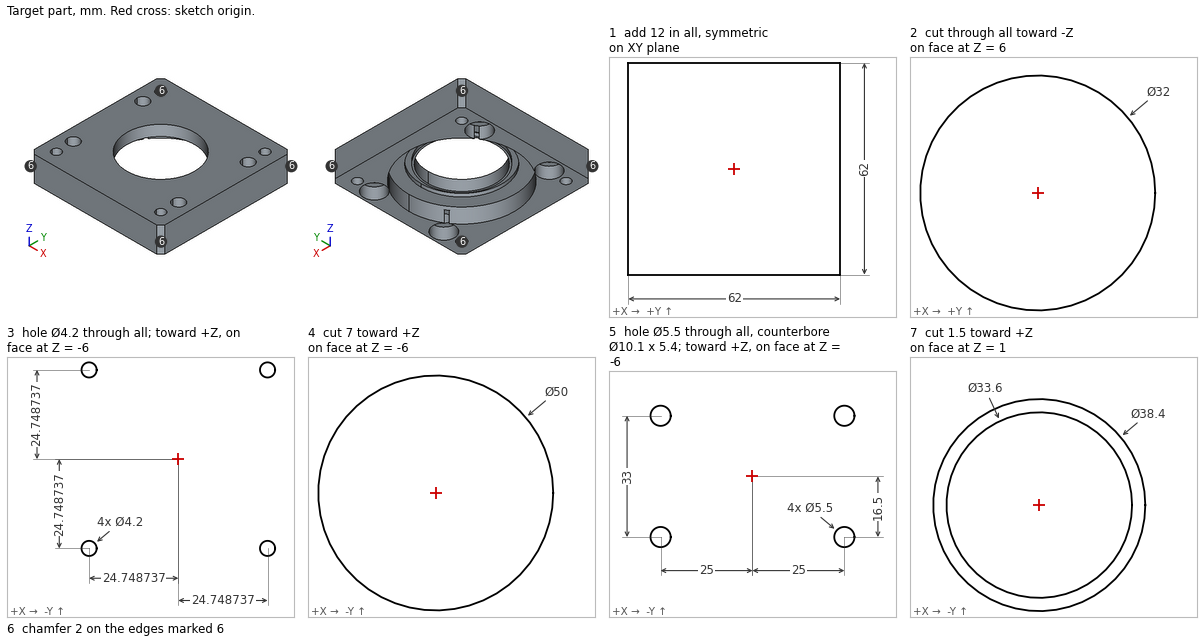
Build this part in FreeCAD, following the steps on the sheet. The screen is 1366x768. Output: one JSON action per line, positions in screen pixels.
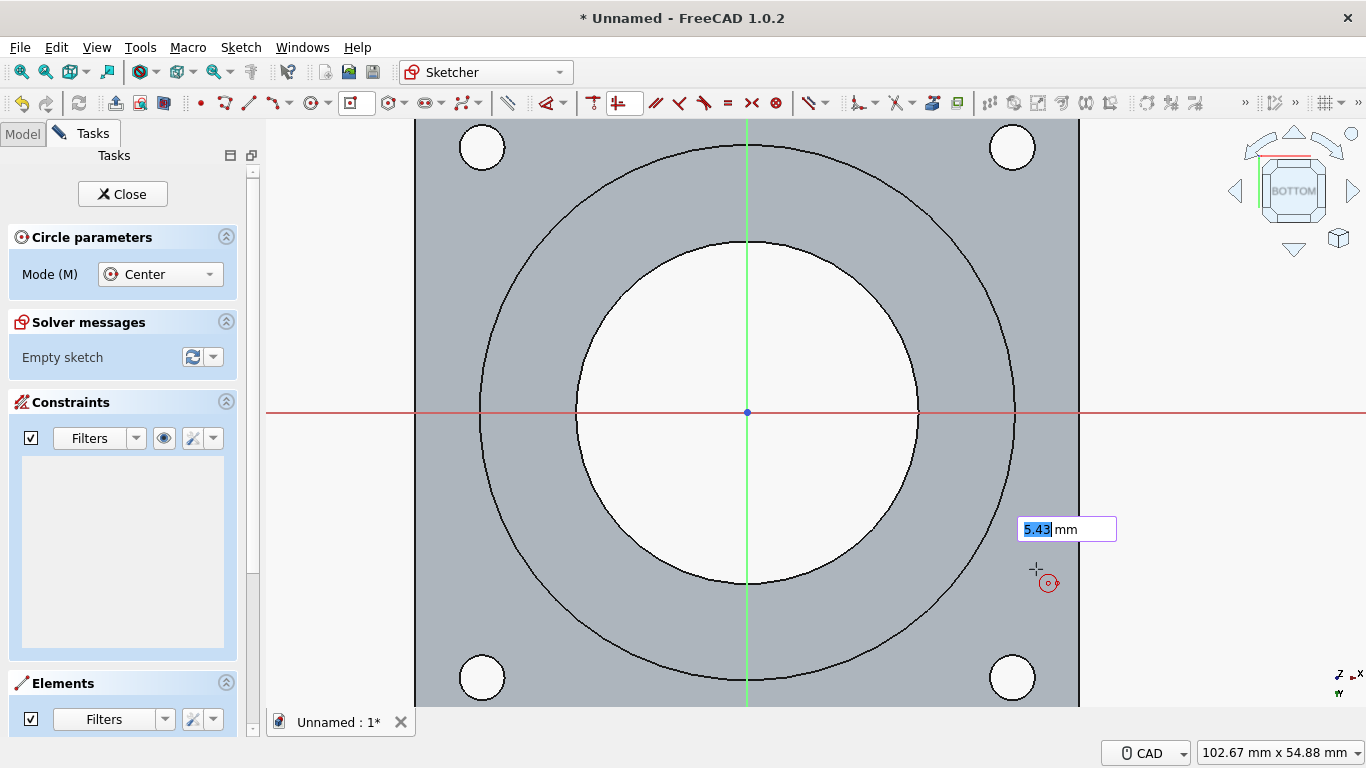
{"action": "type", "text": "5.5"}
{"action": "key", "text": "Return"}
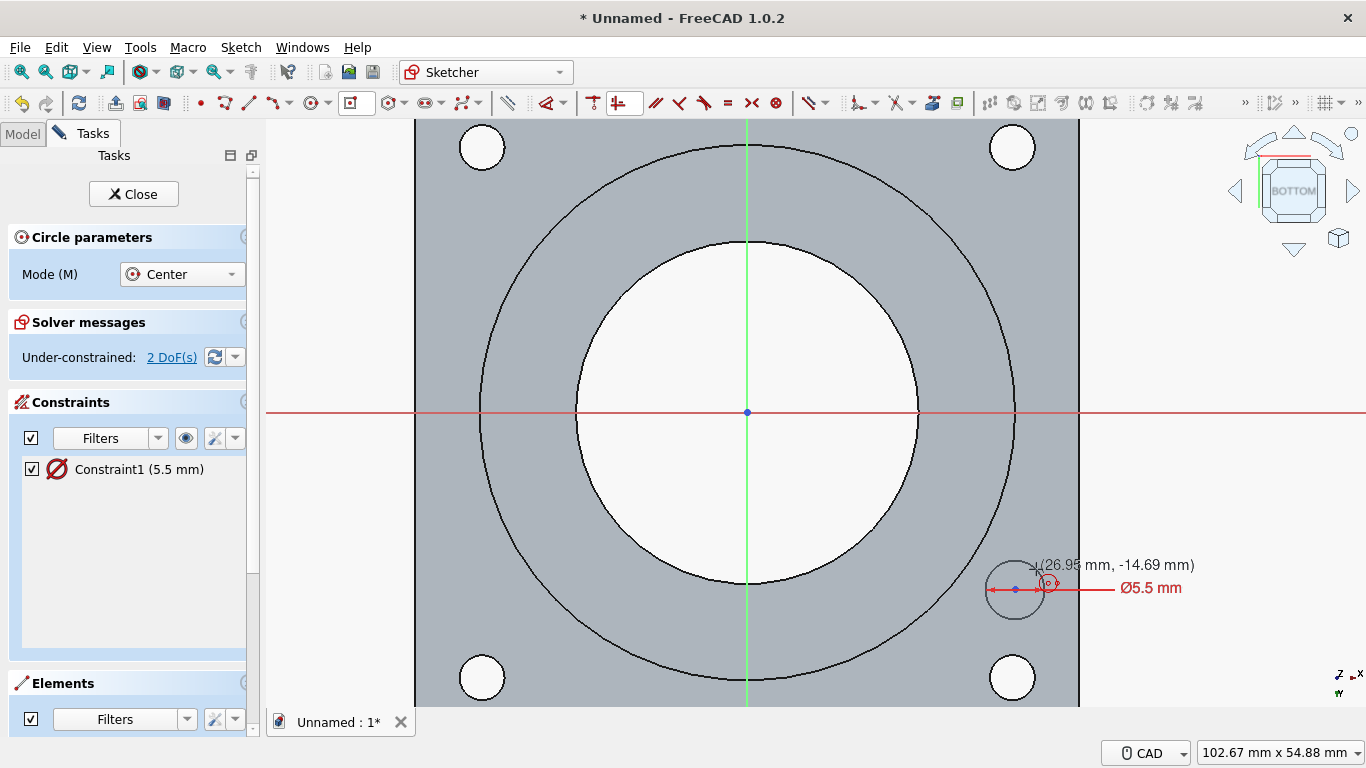
{"action": "left_click", "coordinate": [479, 589]}
{"action": "mouse_move", "coordinate": [500, 569]}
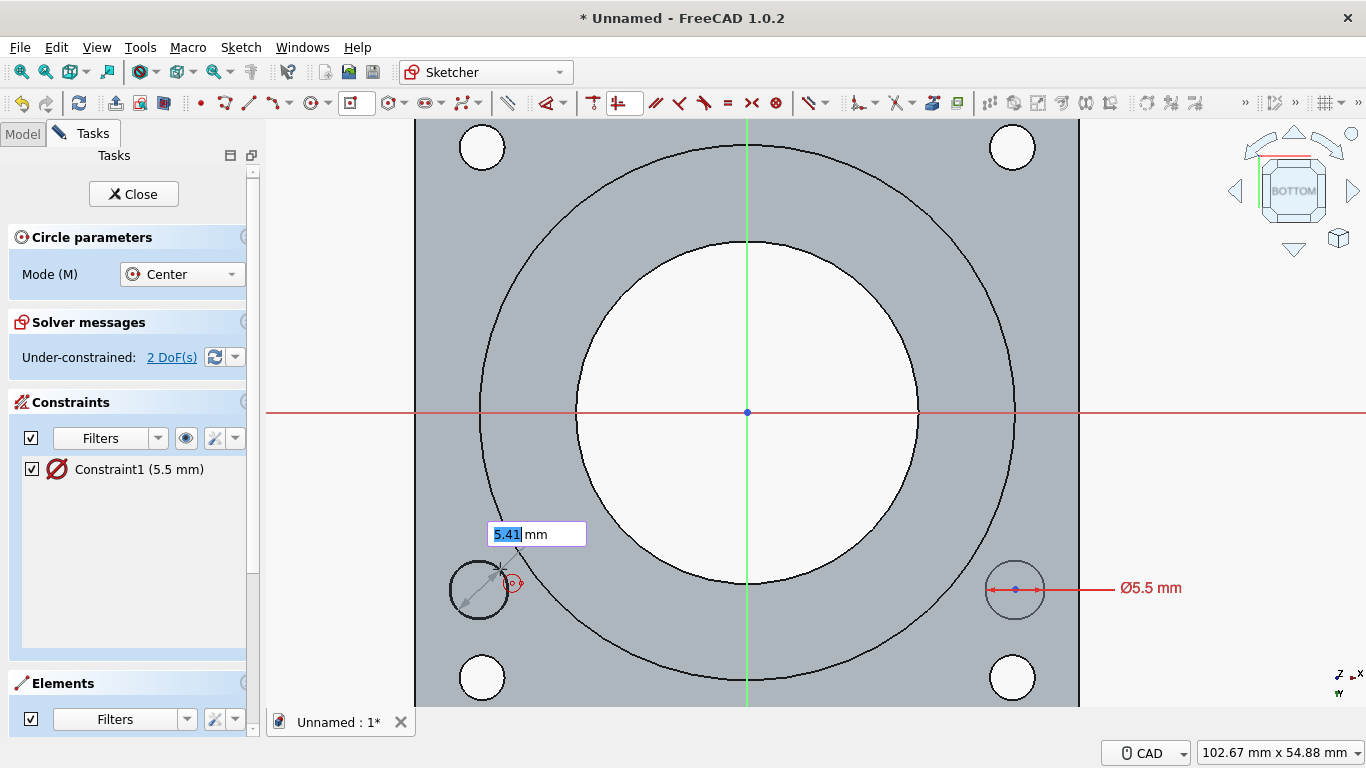
{"action": "type", "text": "5.5"}
{"action": "key", "text": "Return"}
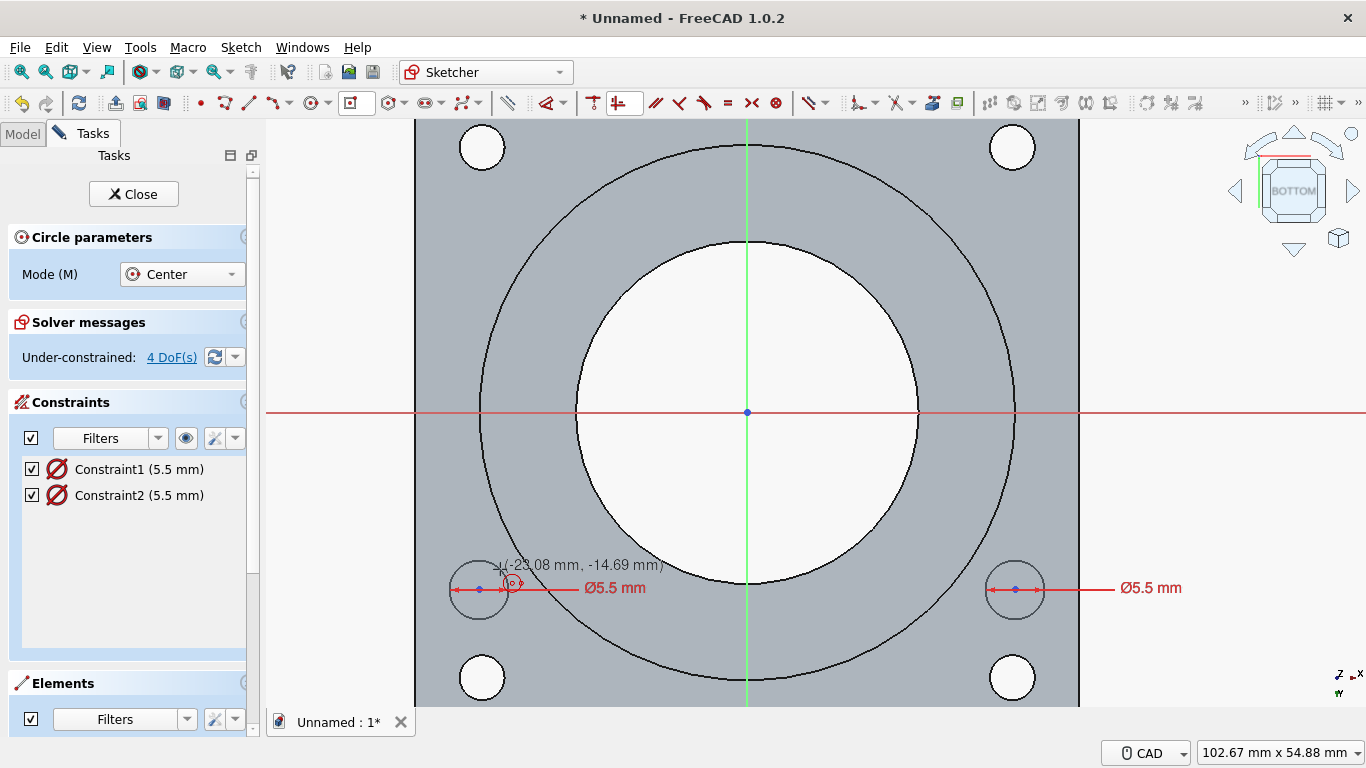
{"action": "left_click", "coordinate": [479, 236]}
{"action": "mouse_move", "coordinate": [500, 215]}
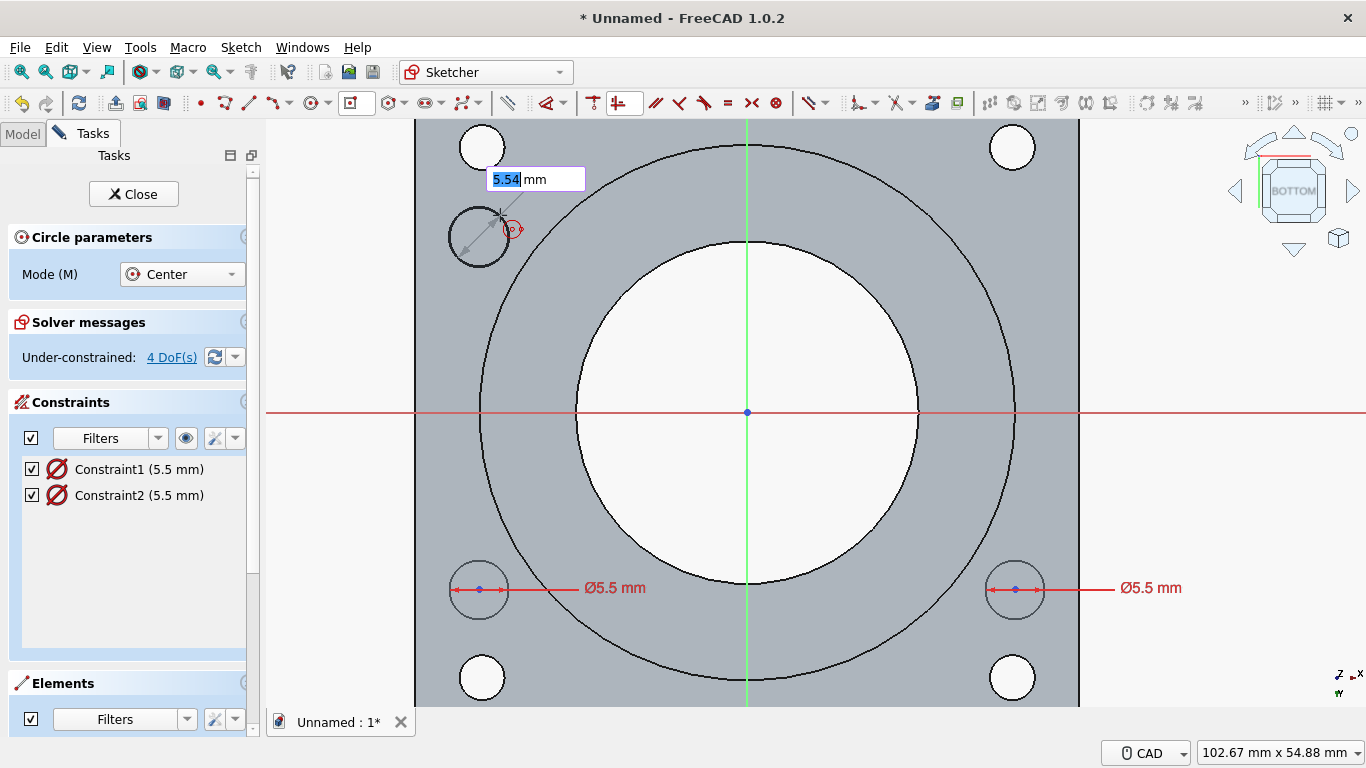
{"action": "type", "text": "5.5"}
{"action": "key", "text": "Return"}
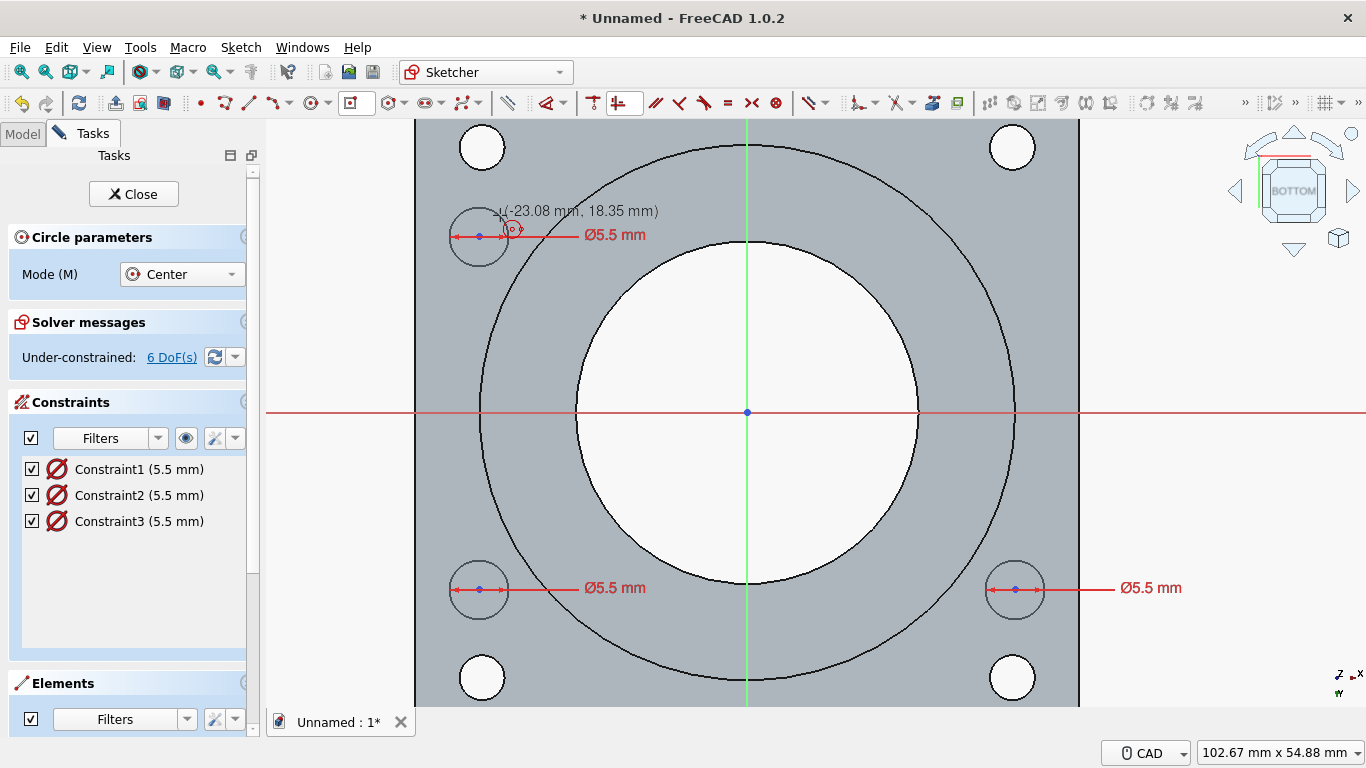
{"action": "left_click", "coordinate": [1015, 236]}
{"action": "mouse_move", "coordinate": [1036, 215]}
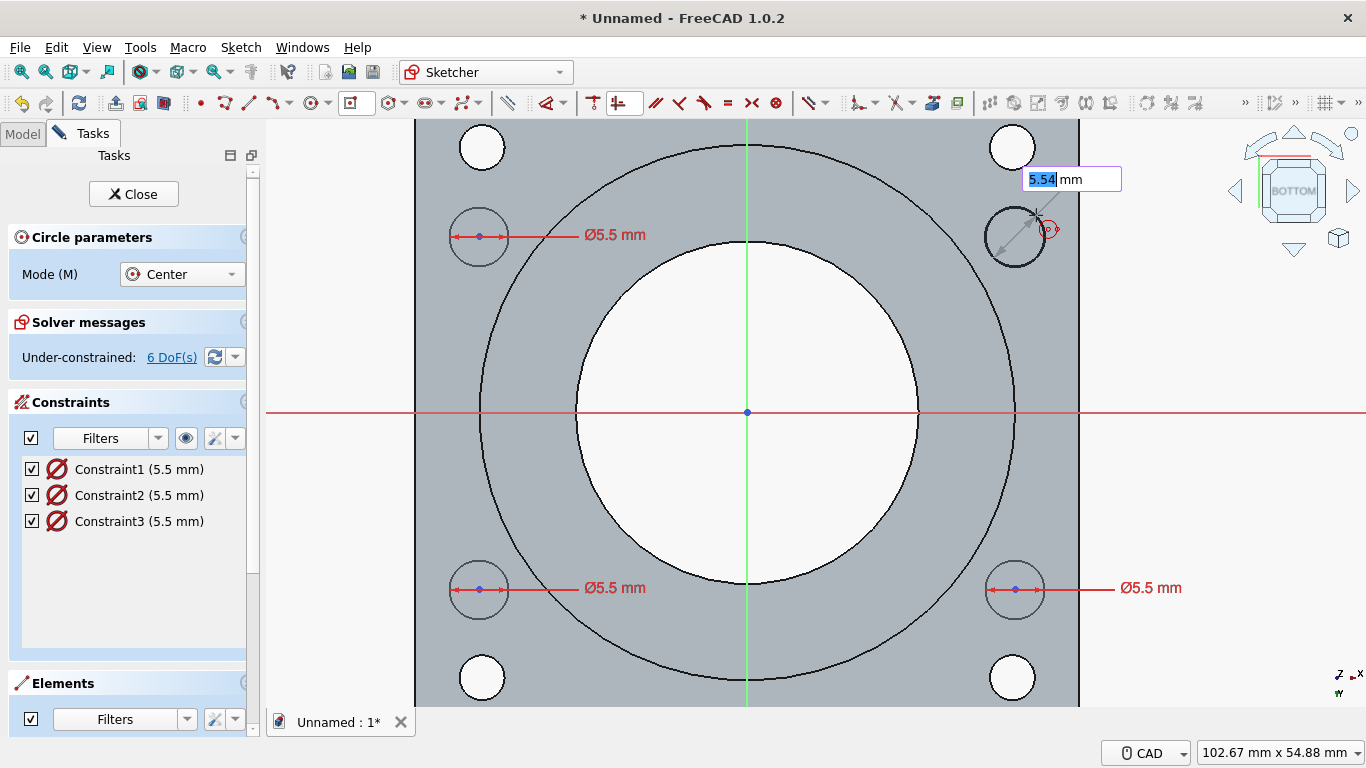
{"action": "type", "text": "5.5"}
{"action": "key", "text": "Return"}
{"action": "key", "text": "Escape"}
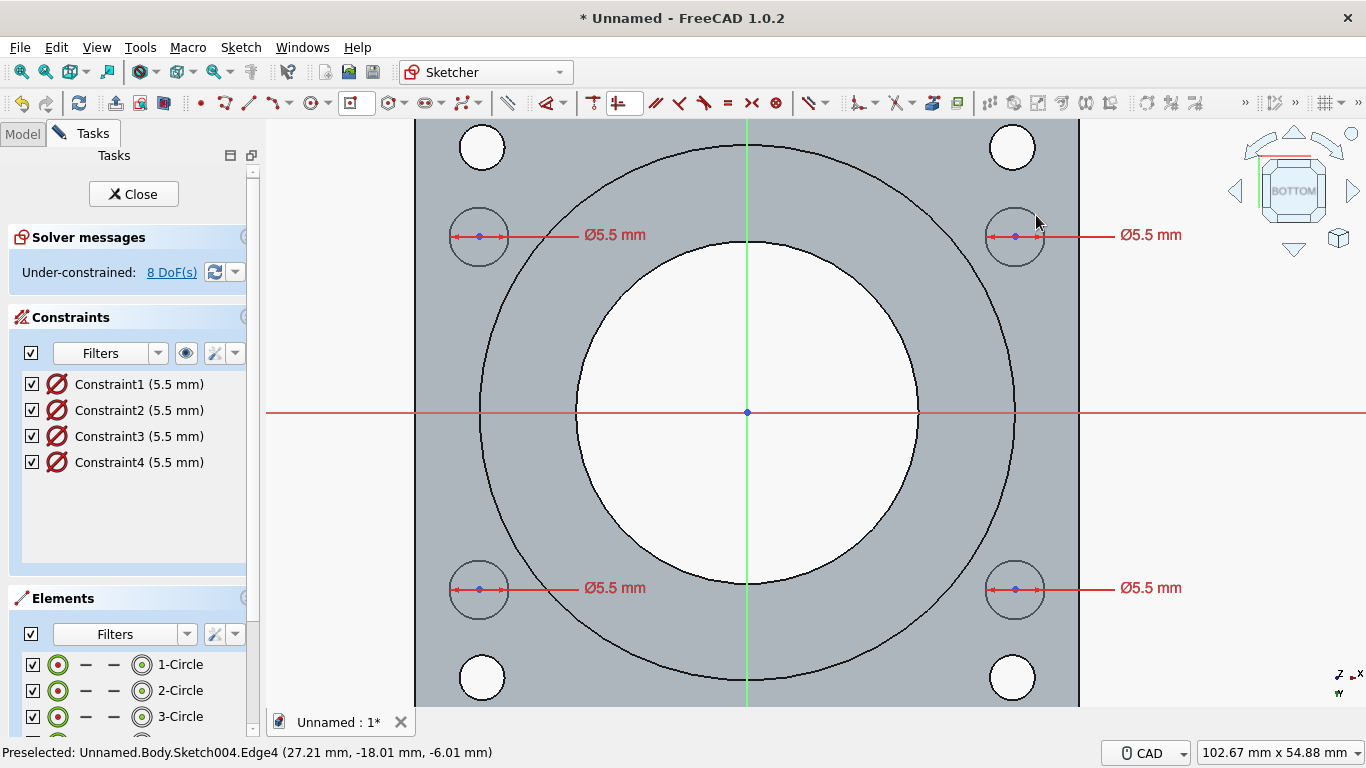
{"action": "left_click", "coordinate": [1015, 590]}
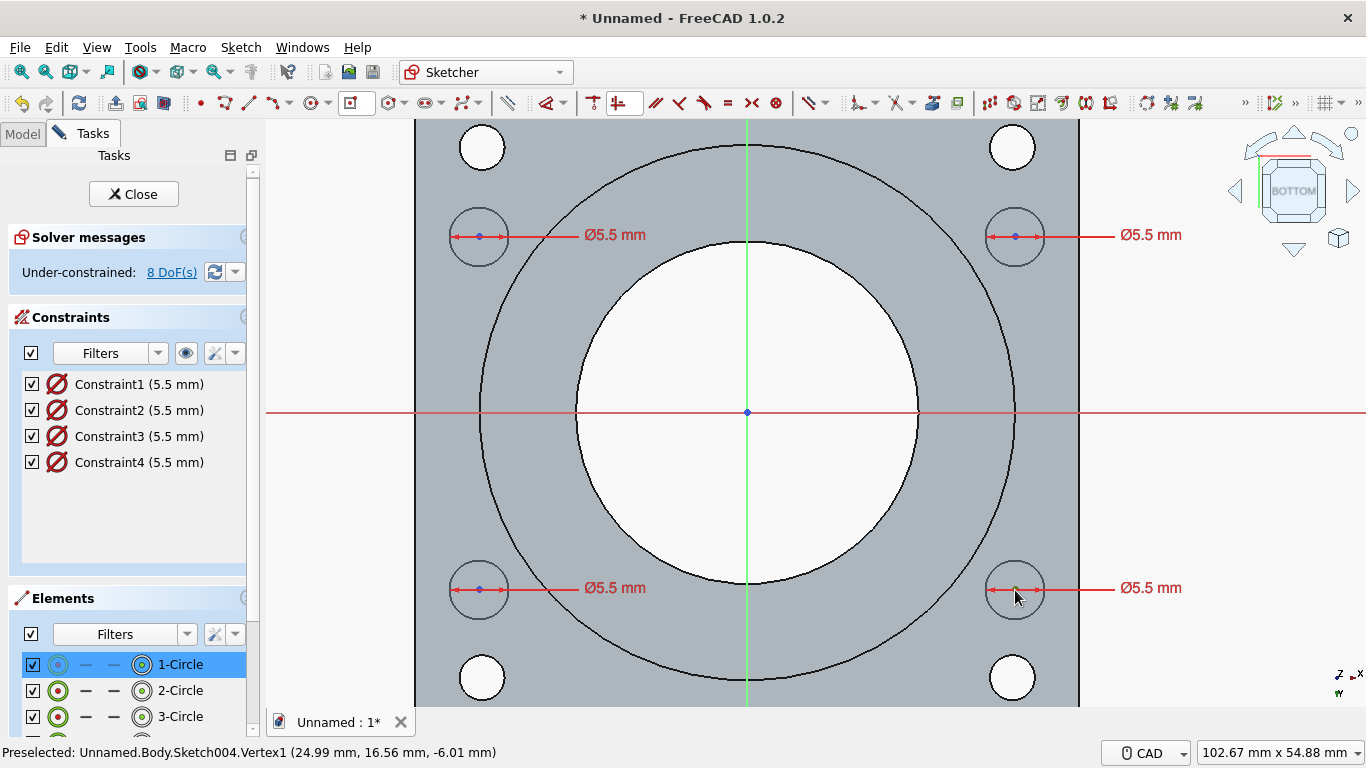
{"action": "left_click", "coordinate": [479, 590]}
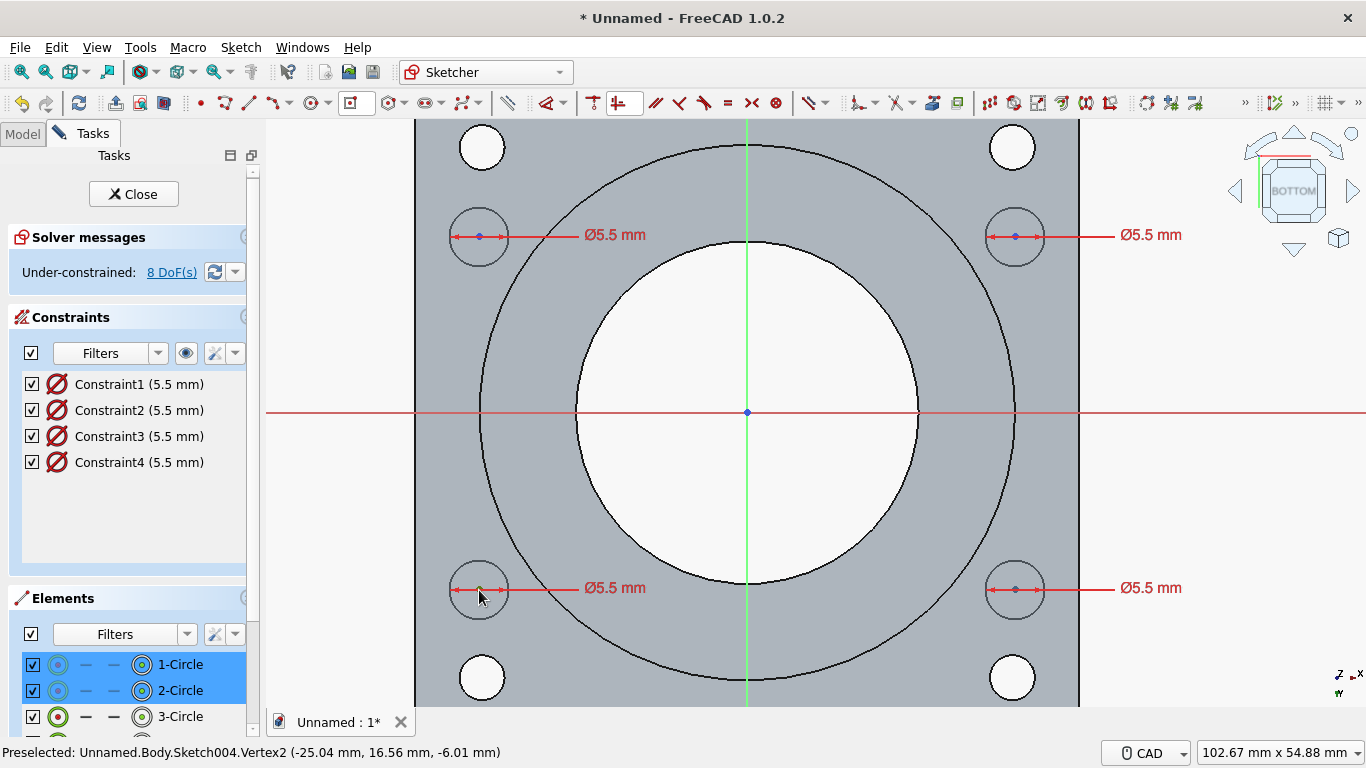
{"action": "left_click", "coordinate": [638, 104]}